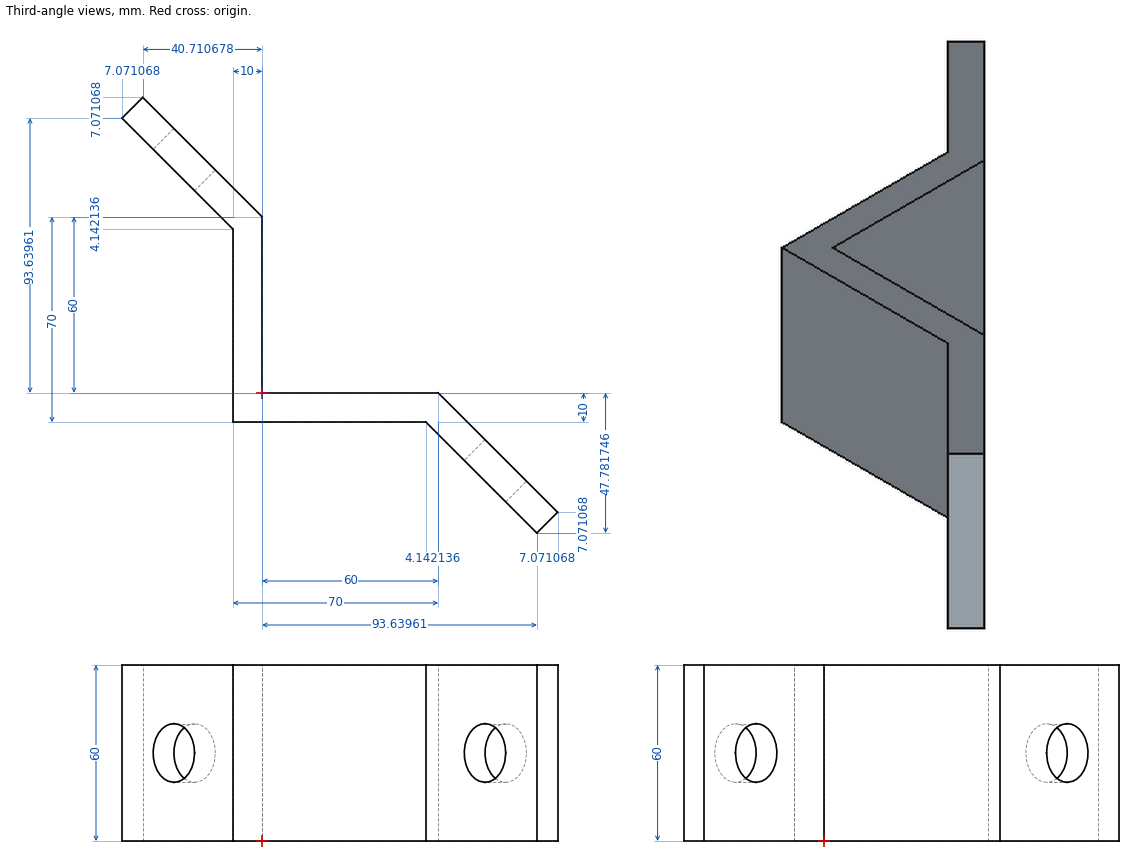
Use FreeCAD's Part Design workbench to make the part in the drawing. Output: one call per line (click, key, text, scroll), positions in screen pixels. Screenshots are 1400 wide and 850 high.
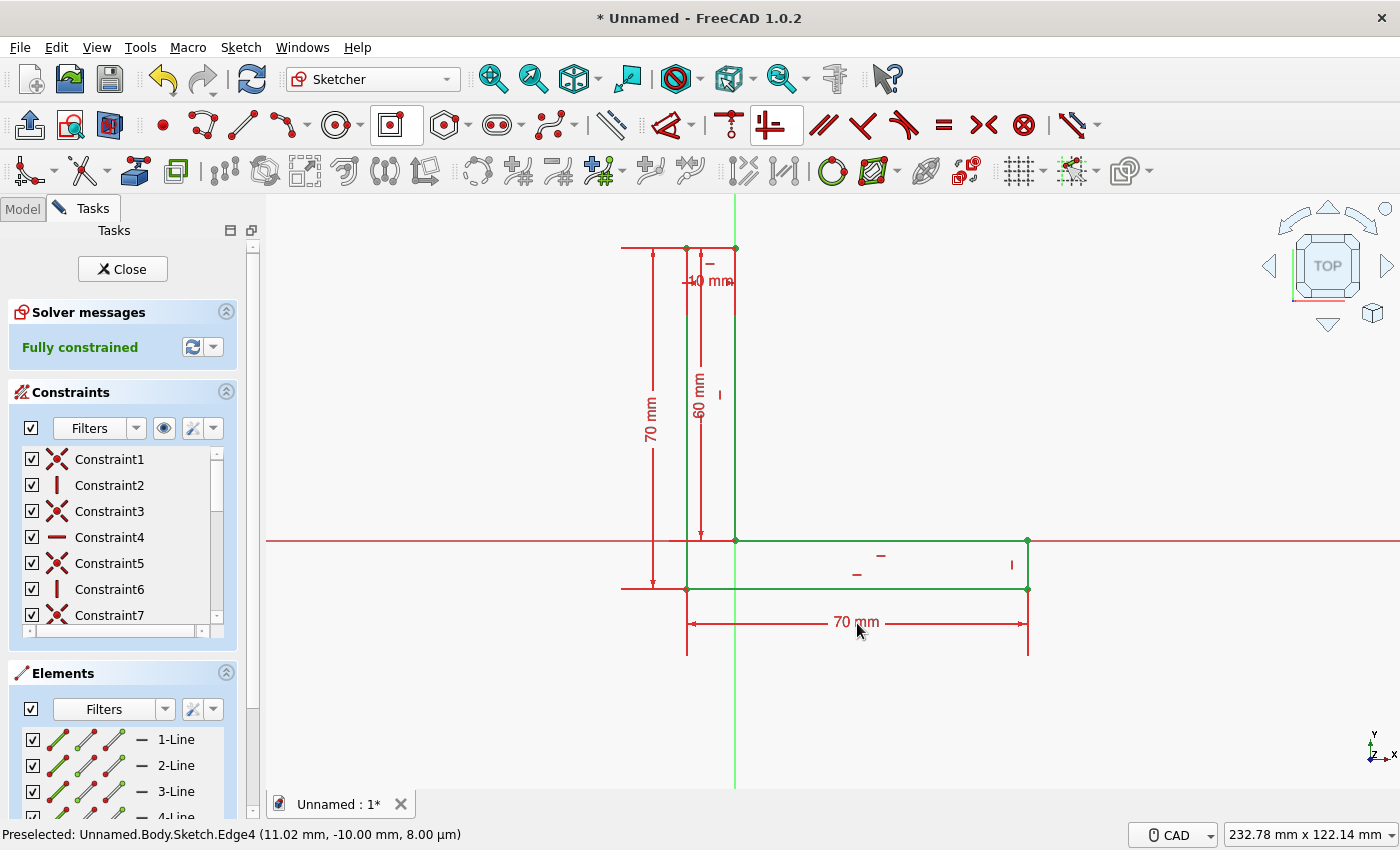
click(123, 269)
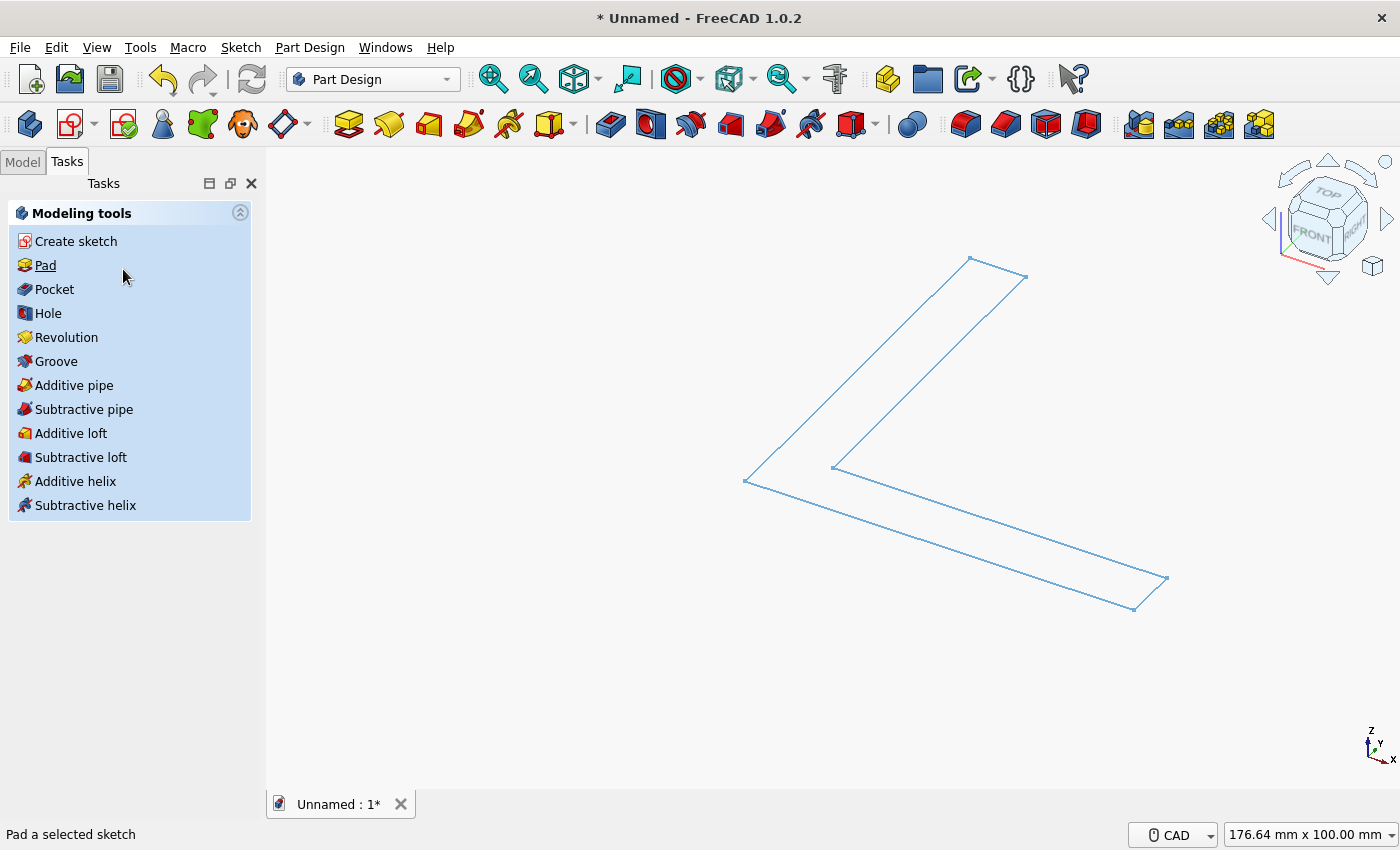
click(350, 124)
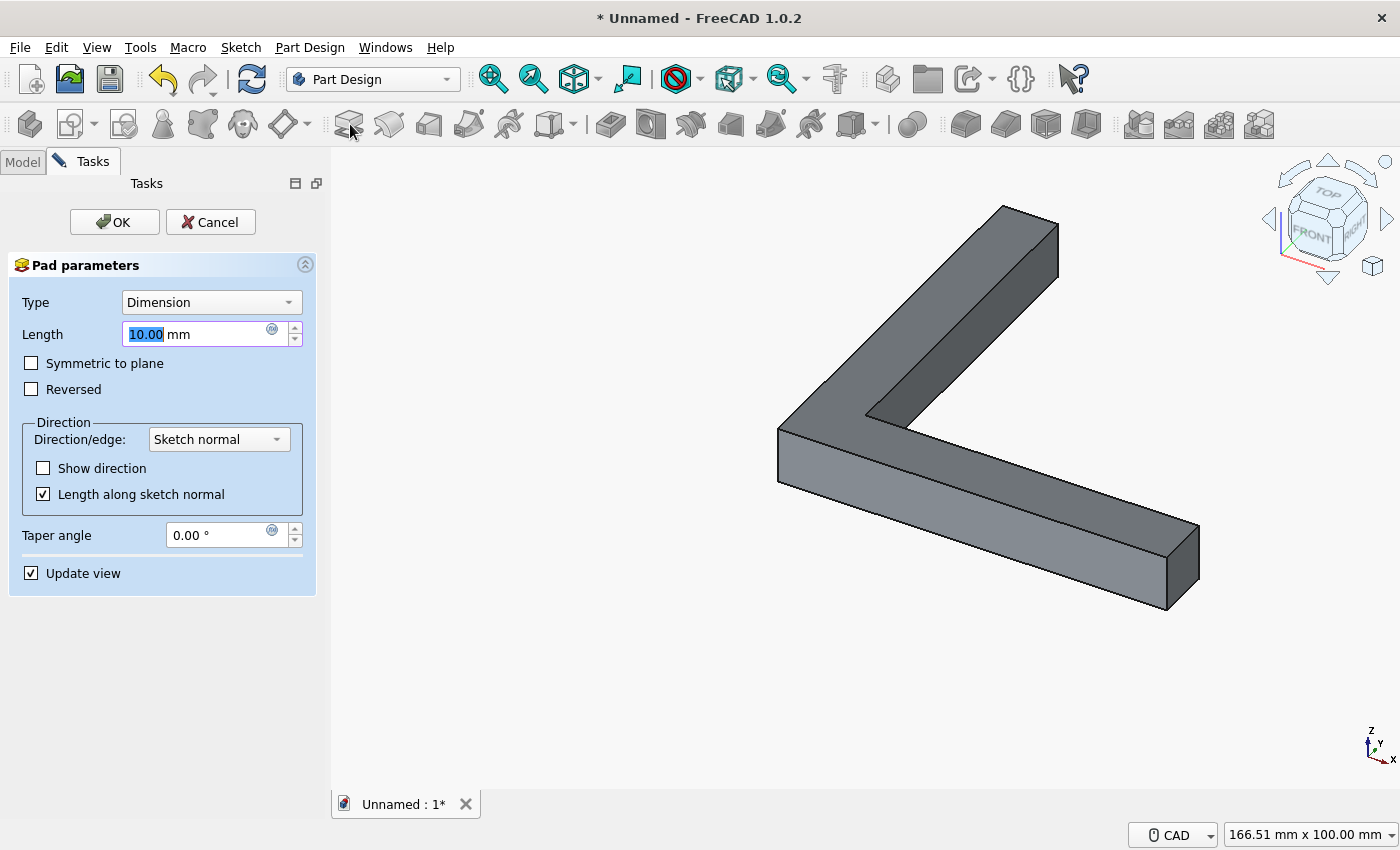
text(60)
key(Tab)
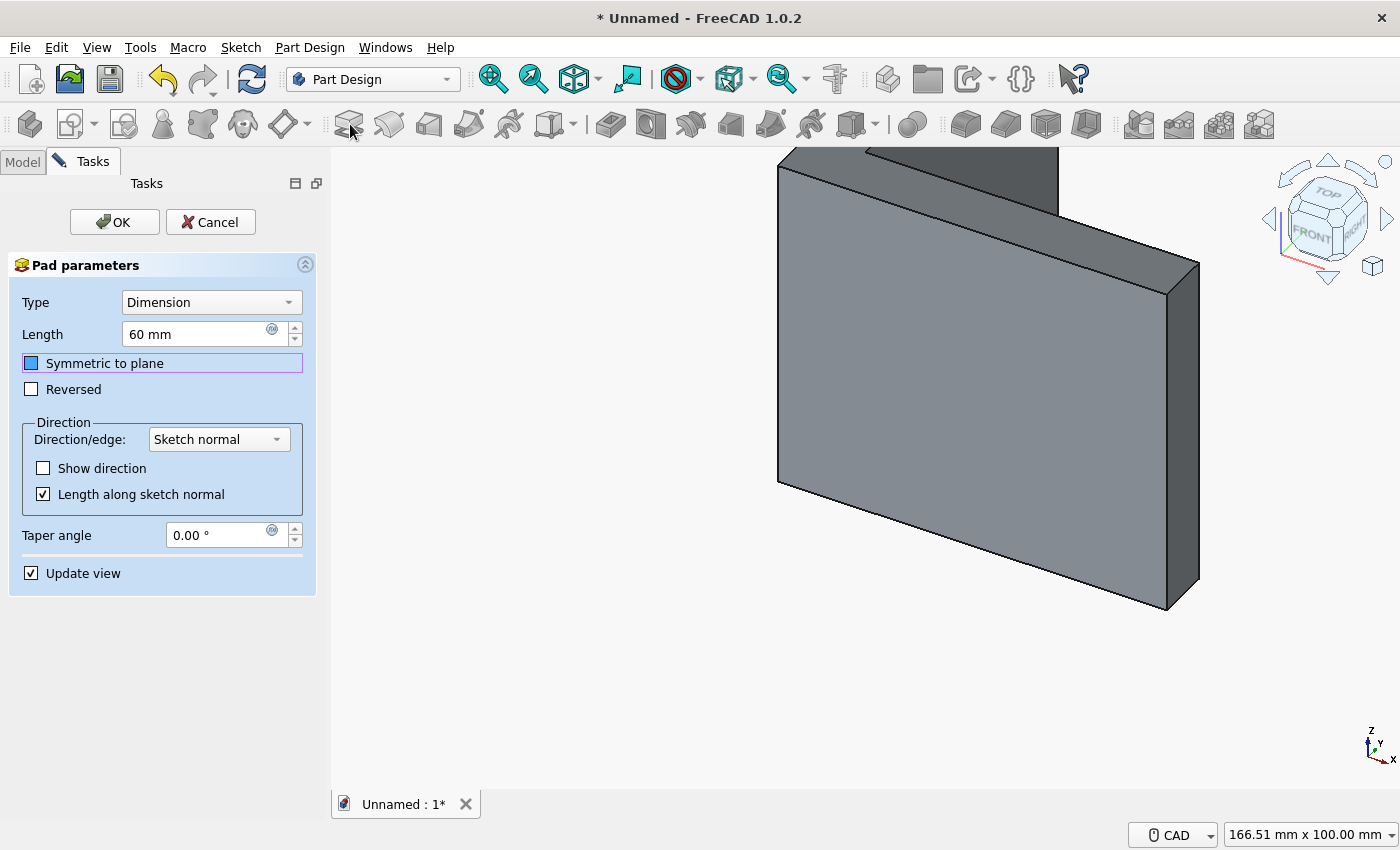
click(115, 222)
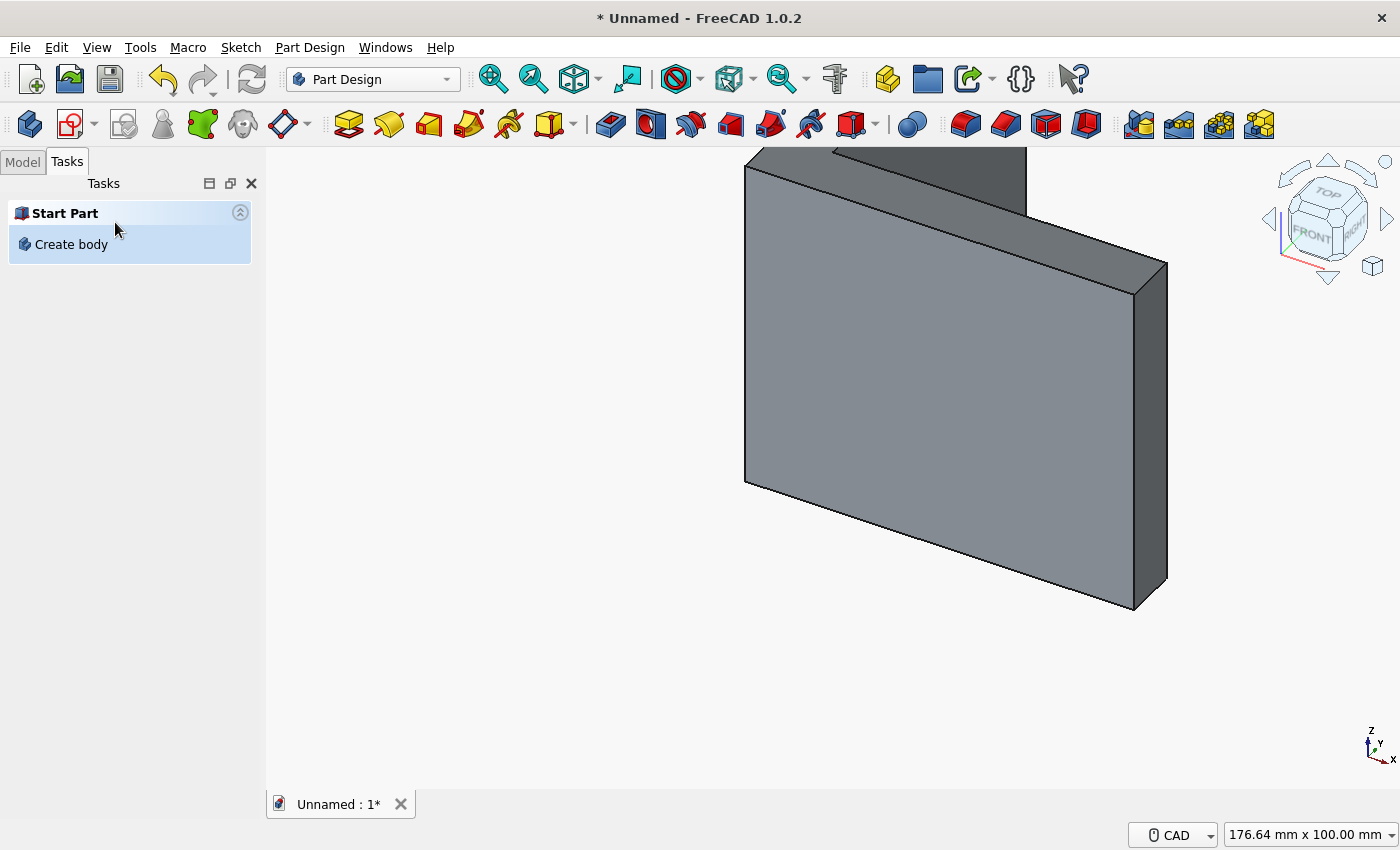
key(v)
key(f)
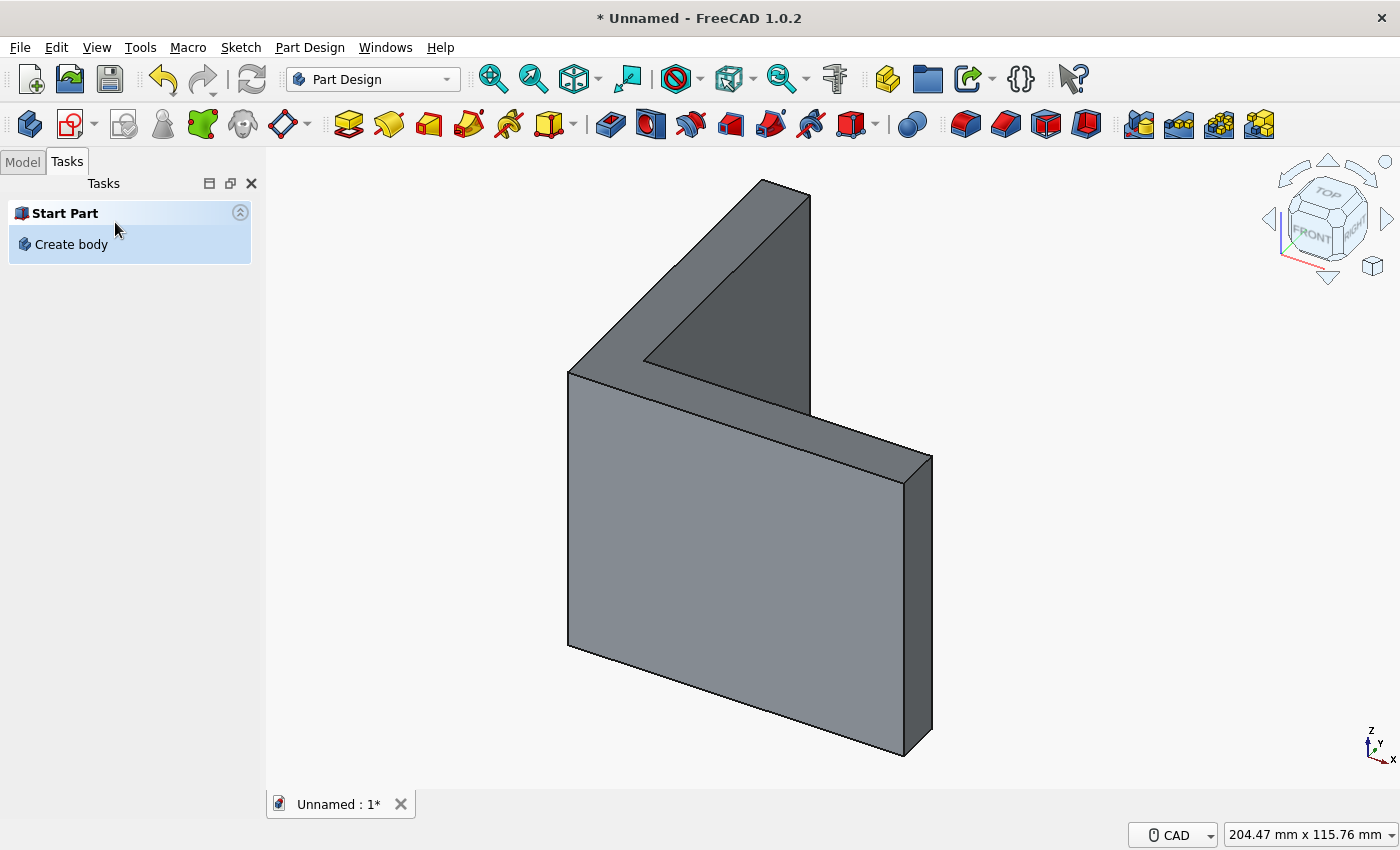
key(5)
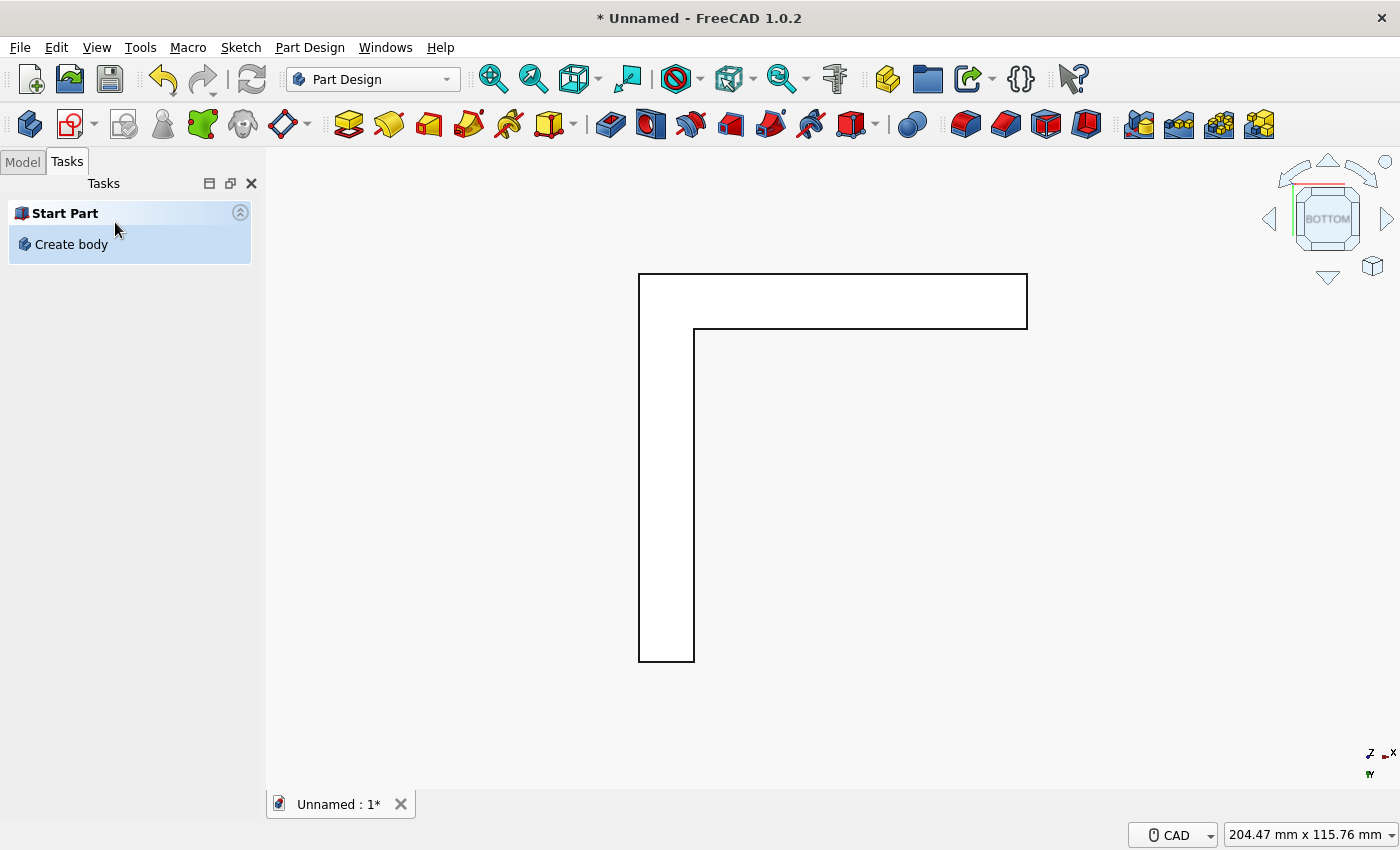
click(999, 301)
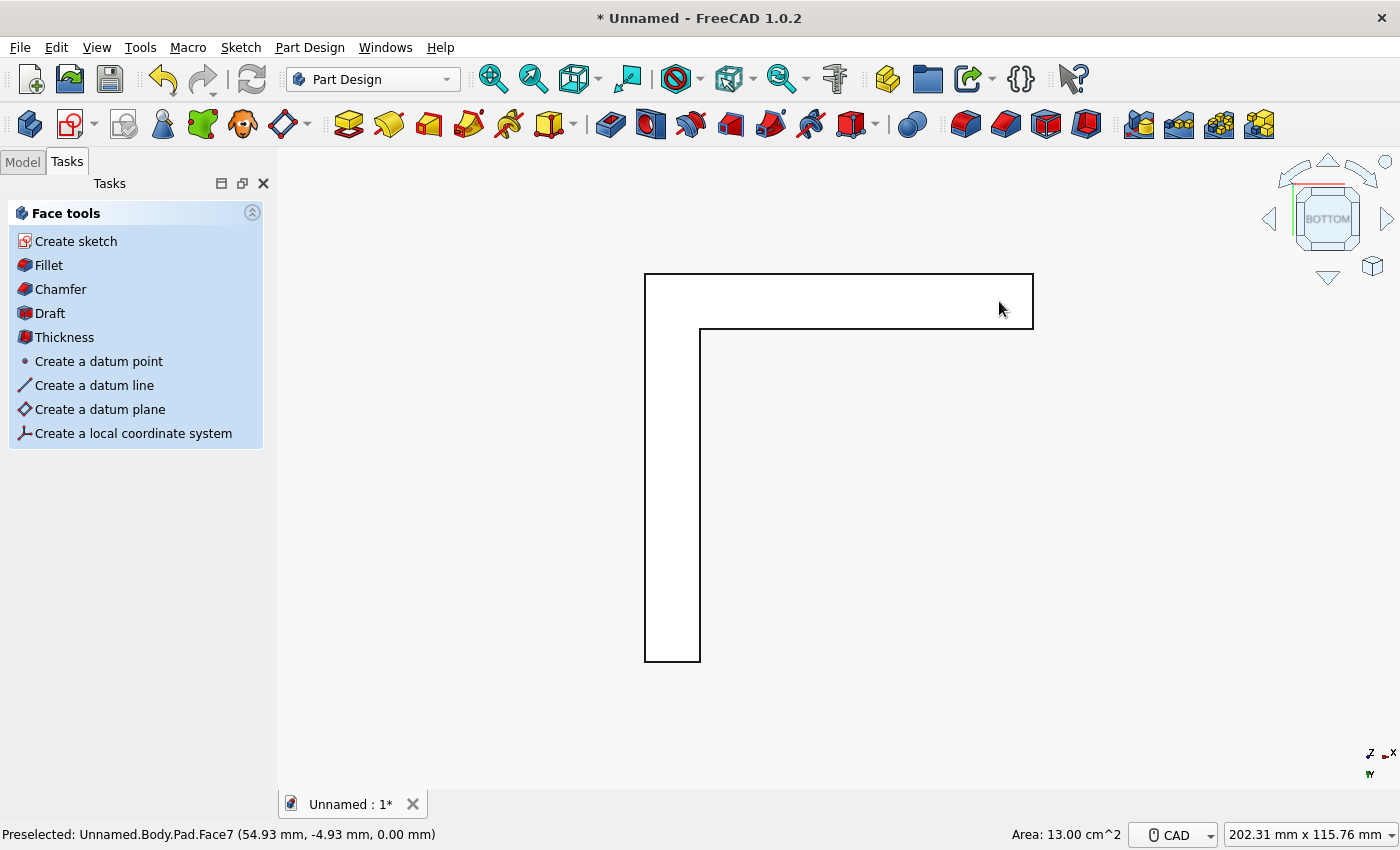
click(70, 124)